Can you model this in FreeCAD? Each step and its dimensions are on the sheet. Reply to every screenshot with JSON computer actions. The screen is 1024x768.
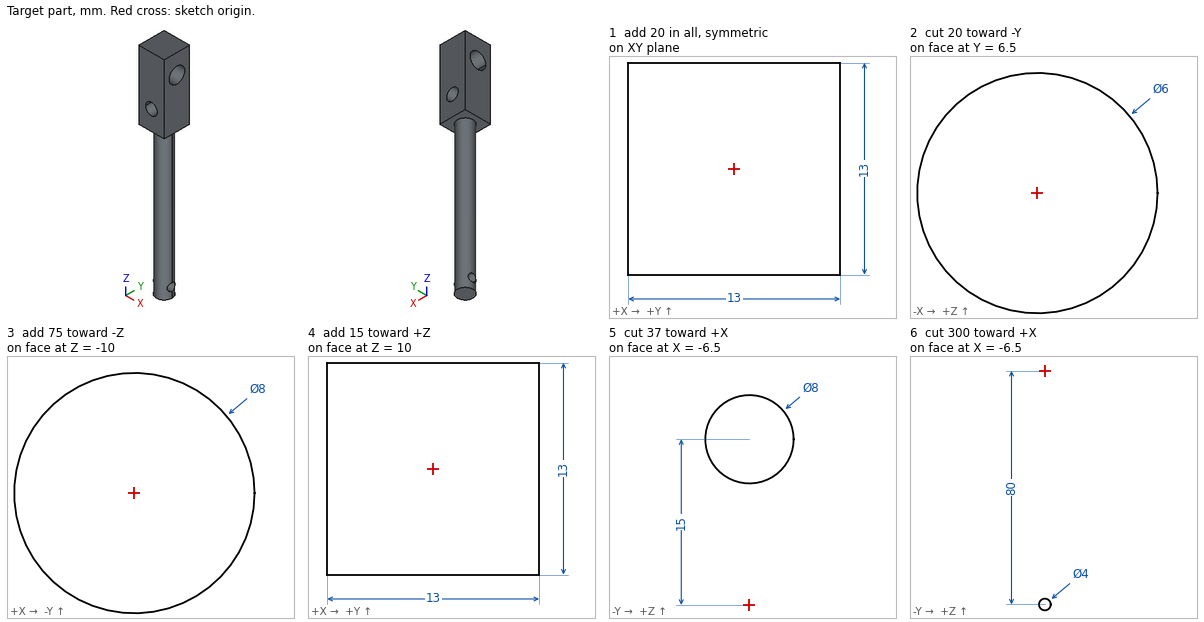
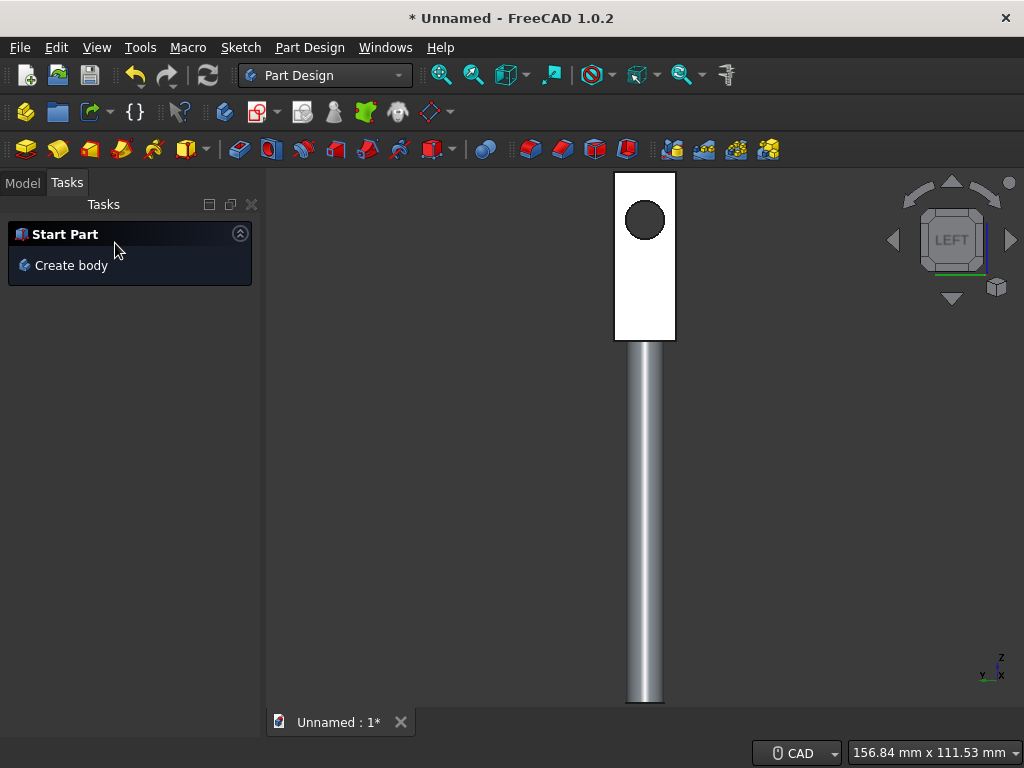
{"action": "left_click", "coordinate": [645, 279]}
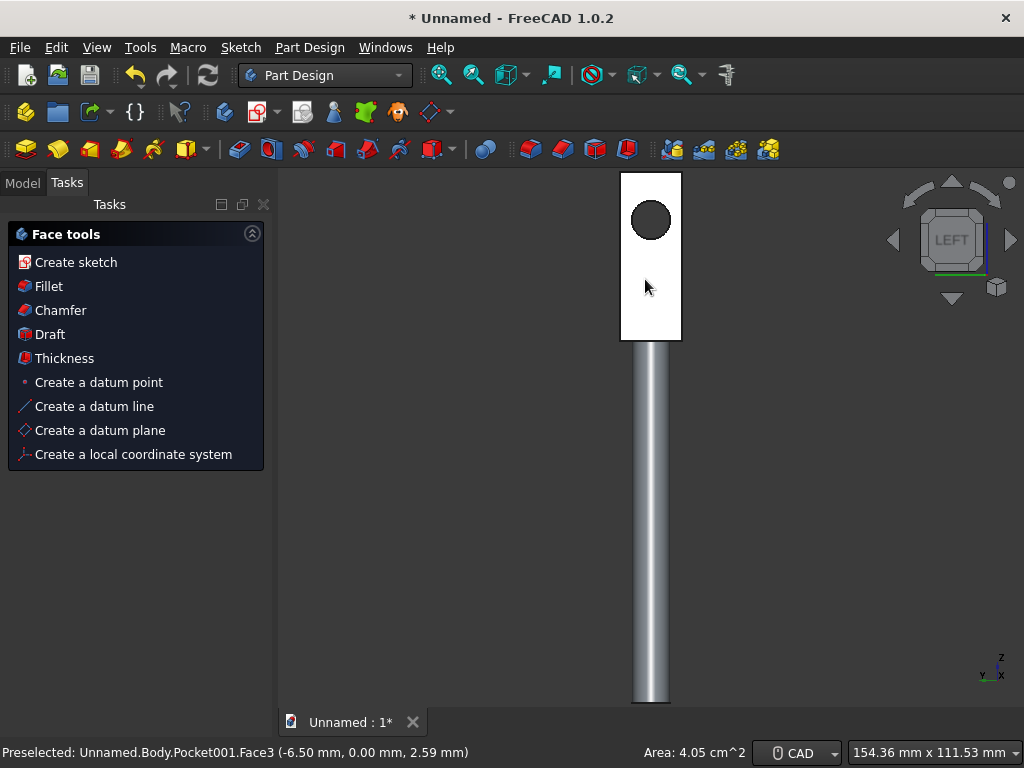
{"action": "left_click", "coordinate": [258, 112]}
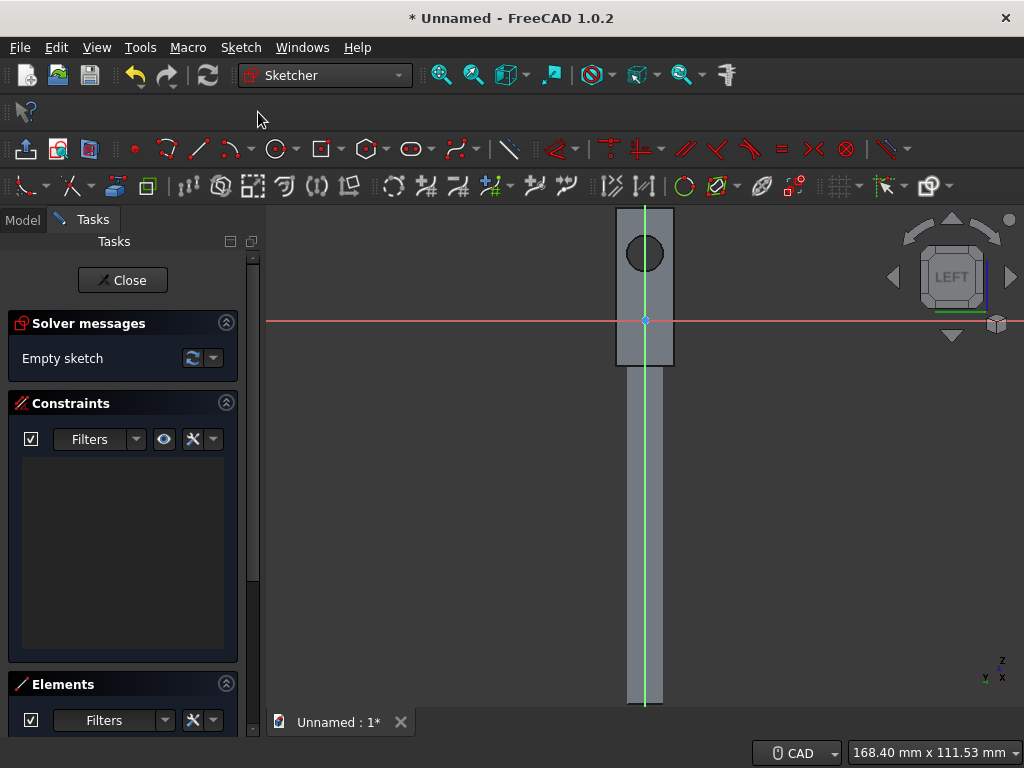
{"action": "scroll", "coordinate": [576, 456], "scroll_direction": "down", "scroll_amount": 5}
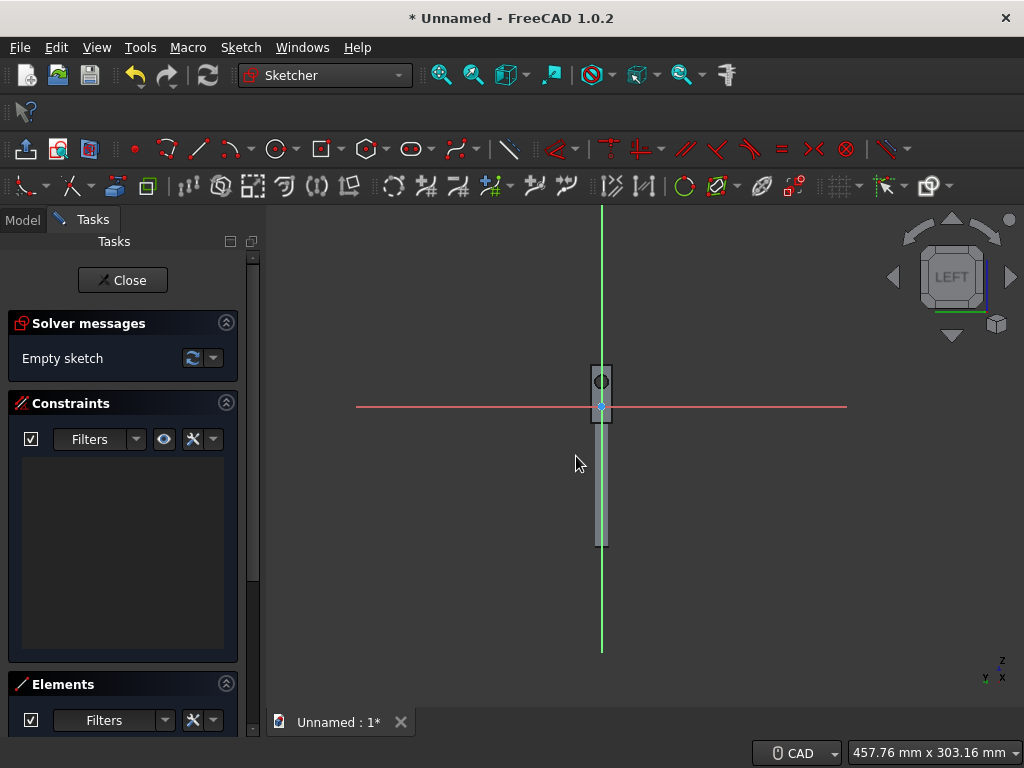
{"action": "scroll", "coordinate": [603, 543], "scroll_direction": "up", "scroll_amount": 15}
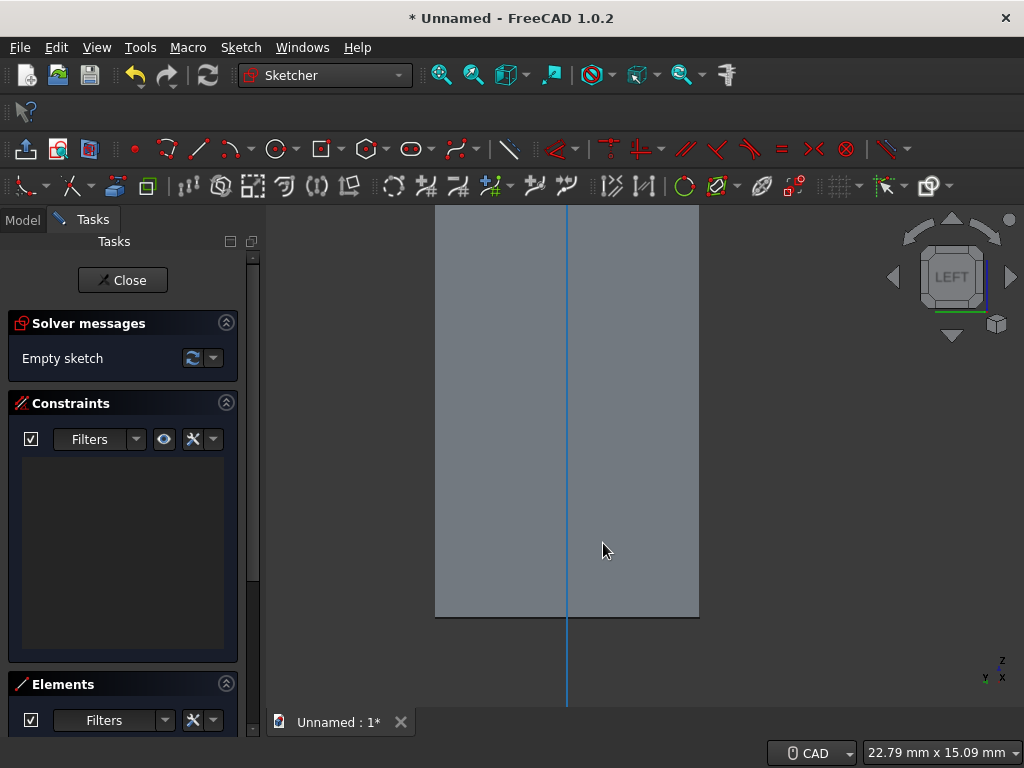
{"action": "scroll", "coordinate": [560, 449], "scroll_direction": "up", "scroll_amount": 4}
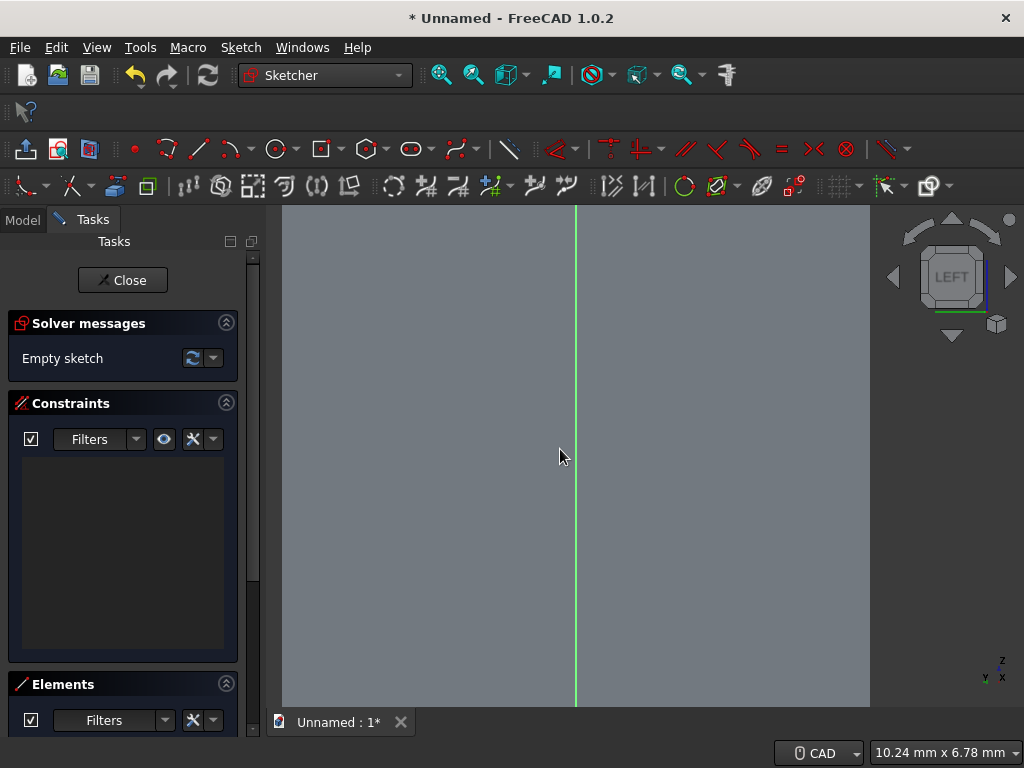
{"action": "key", "text": "g c"}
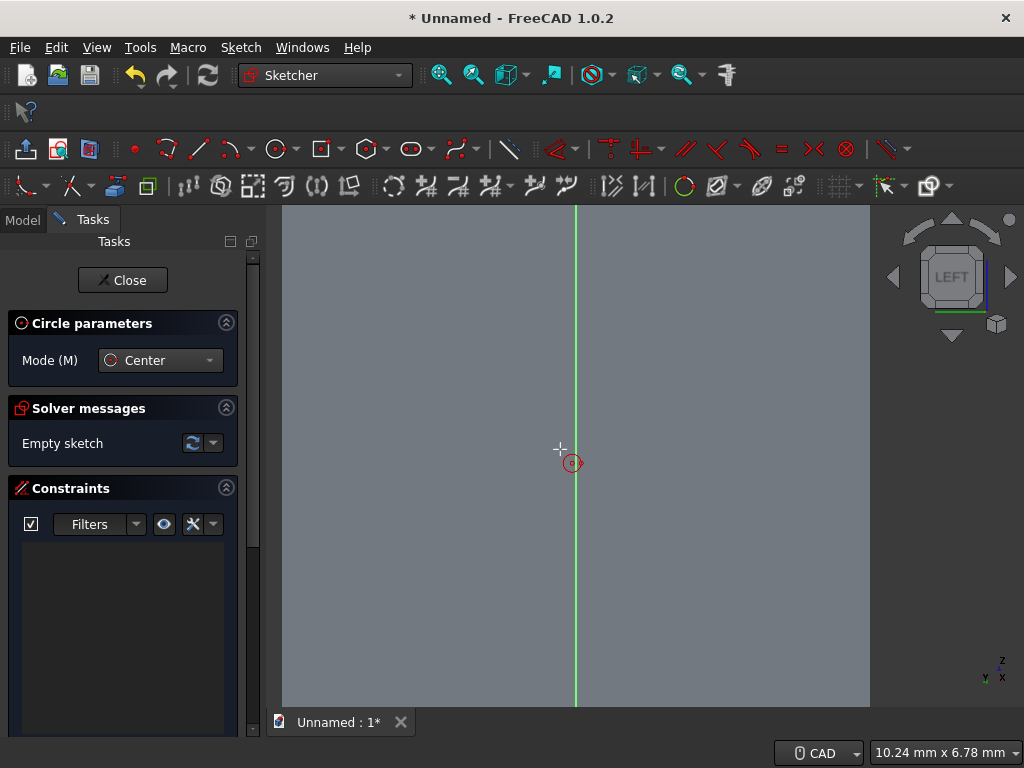
{"action": "left_click", "coordinate": [576, 455]}
{"action": "mouse_move", "coordinate": [680, 350]}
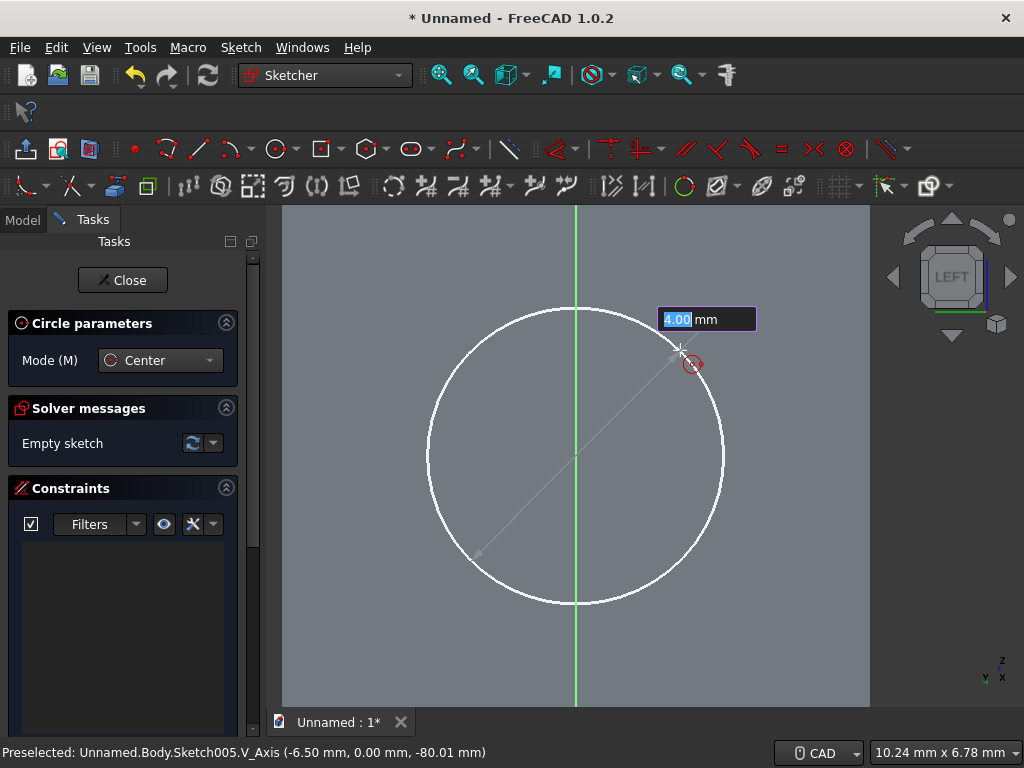
{"action": "type", "text": "4"}
{"action": "key", "text": "Return"}
{"action": "key", "text": "Escape"}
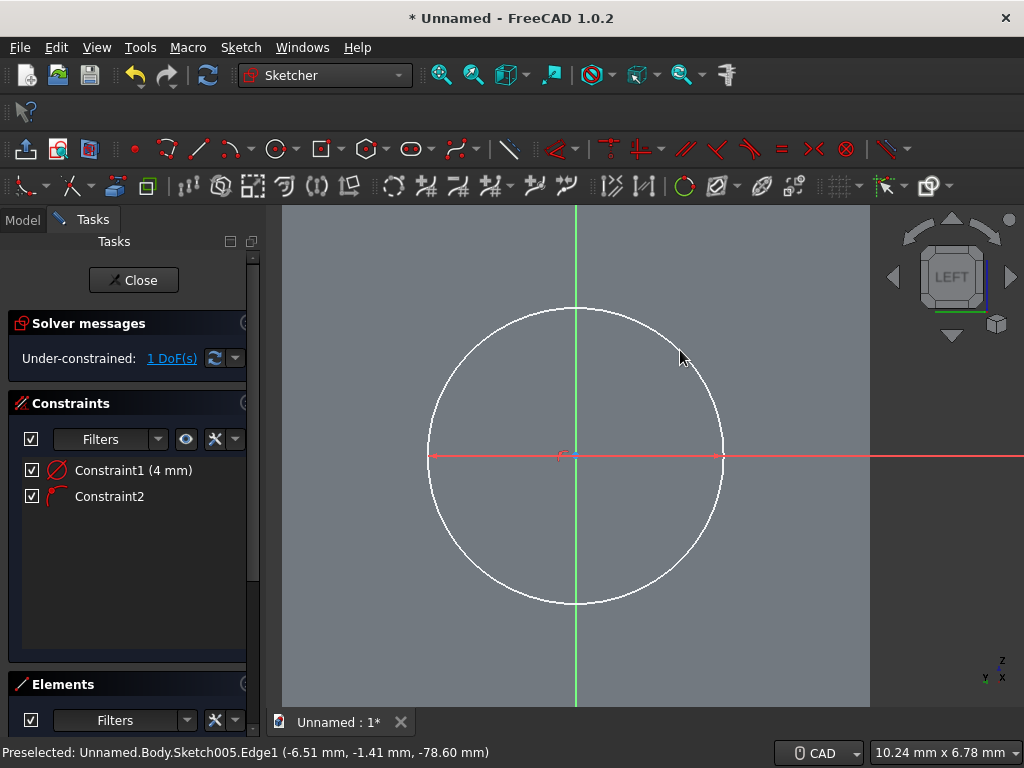
{"action": "left_click", "coordinate": [576, 456]}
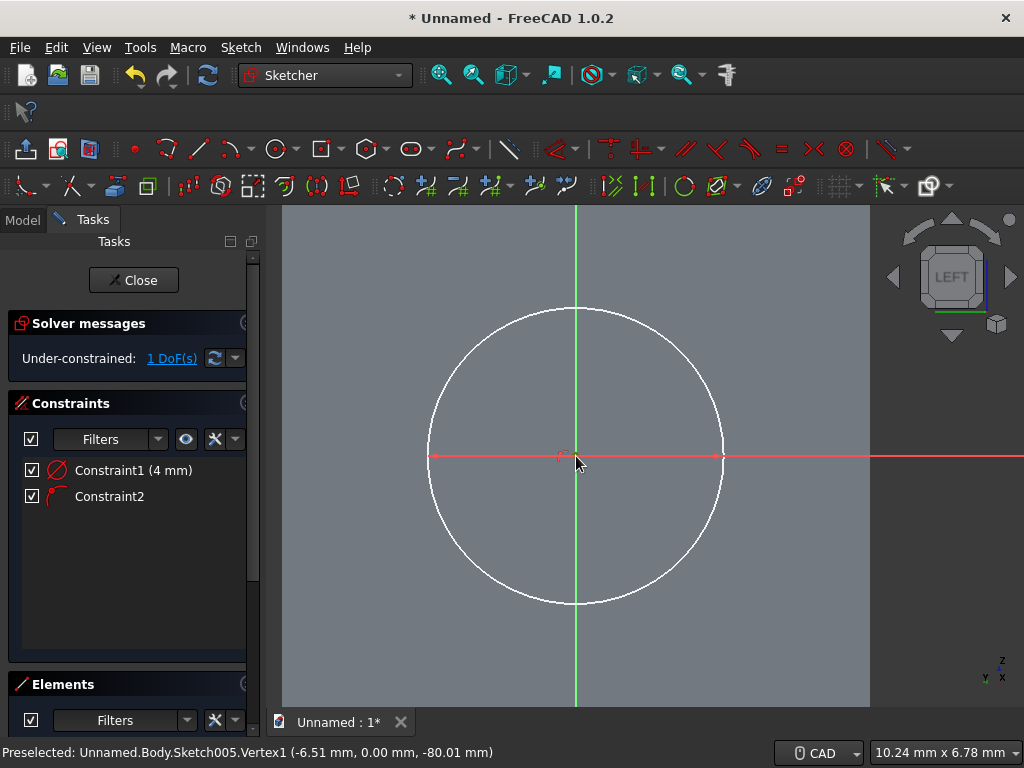
{"action": "key", "text": "i"}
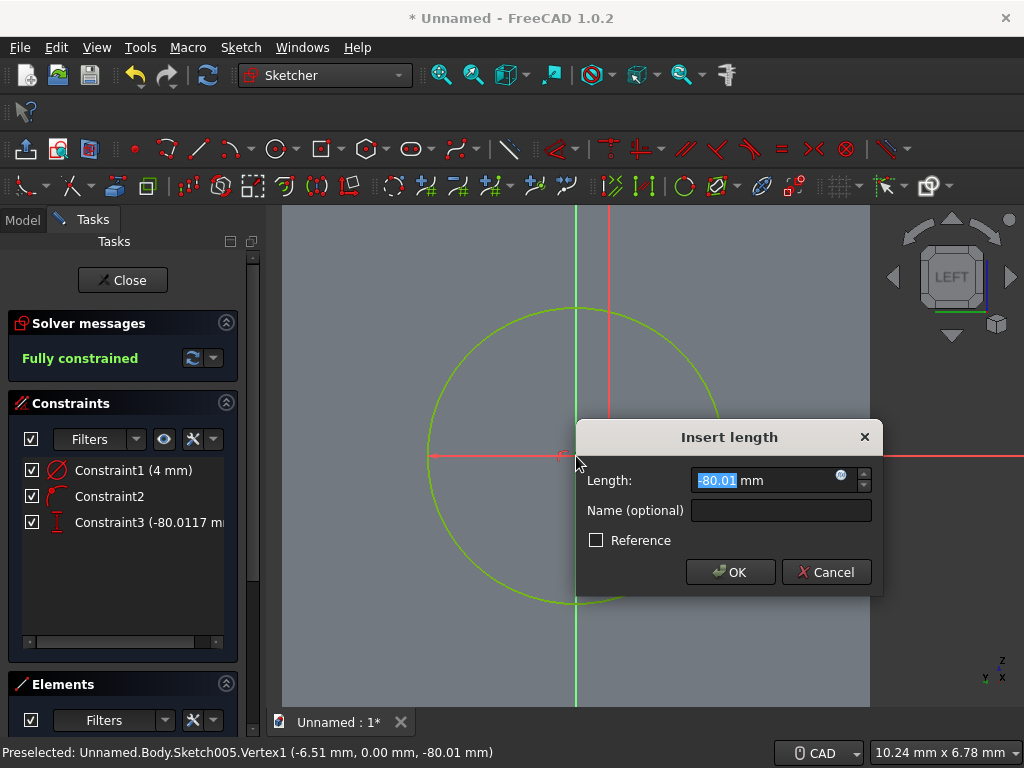
{"action": "type", "text": "-80"}
{"action": "key", "text": "Return"}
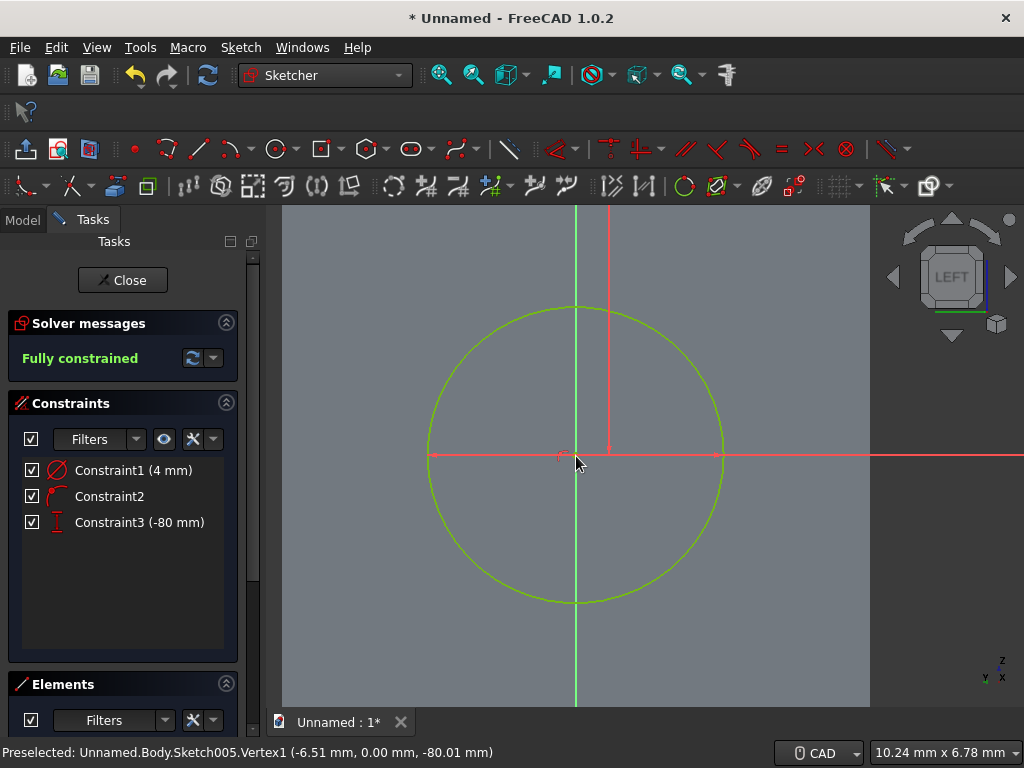
{"action": "left_click", "coordinate": [123, 280]}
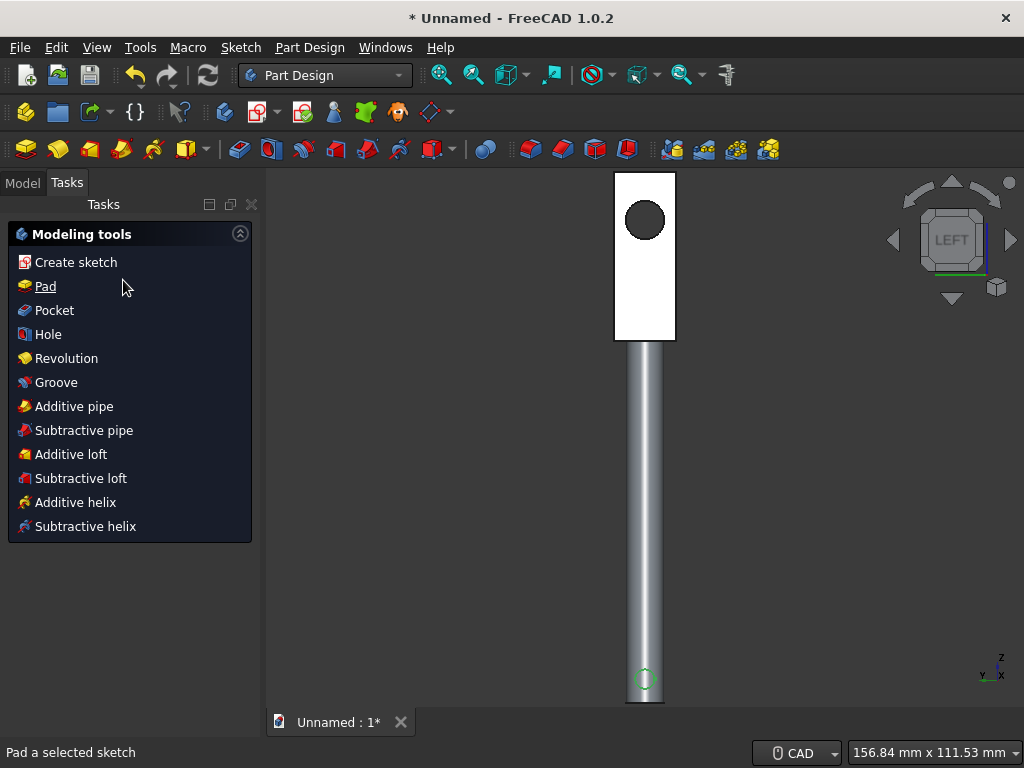
{"action": "left_click", "coordinate": [240, 150]}